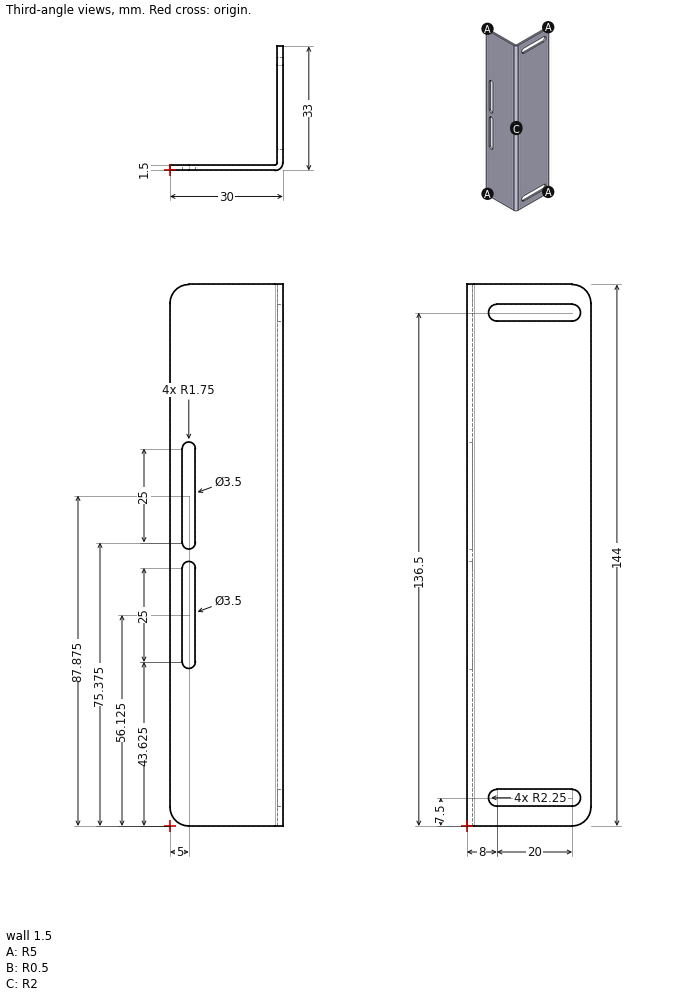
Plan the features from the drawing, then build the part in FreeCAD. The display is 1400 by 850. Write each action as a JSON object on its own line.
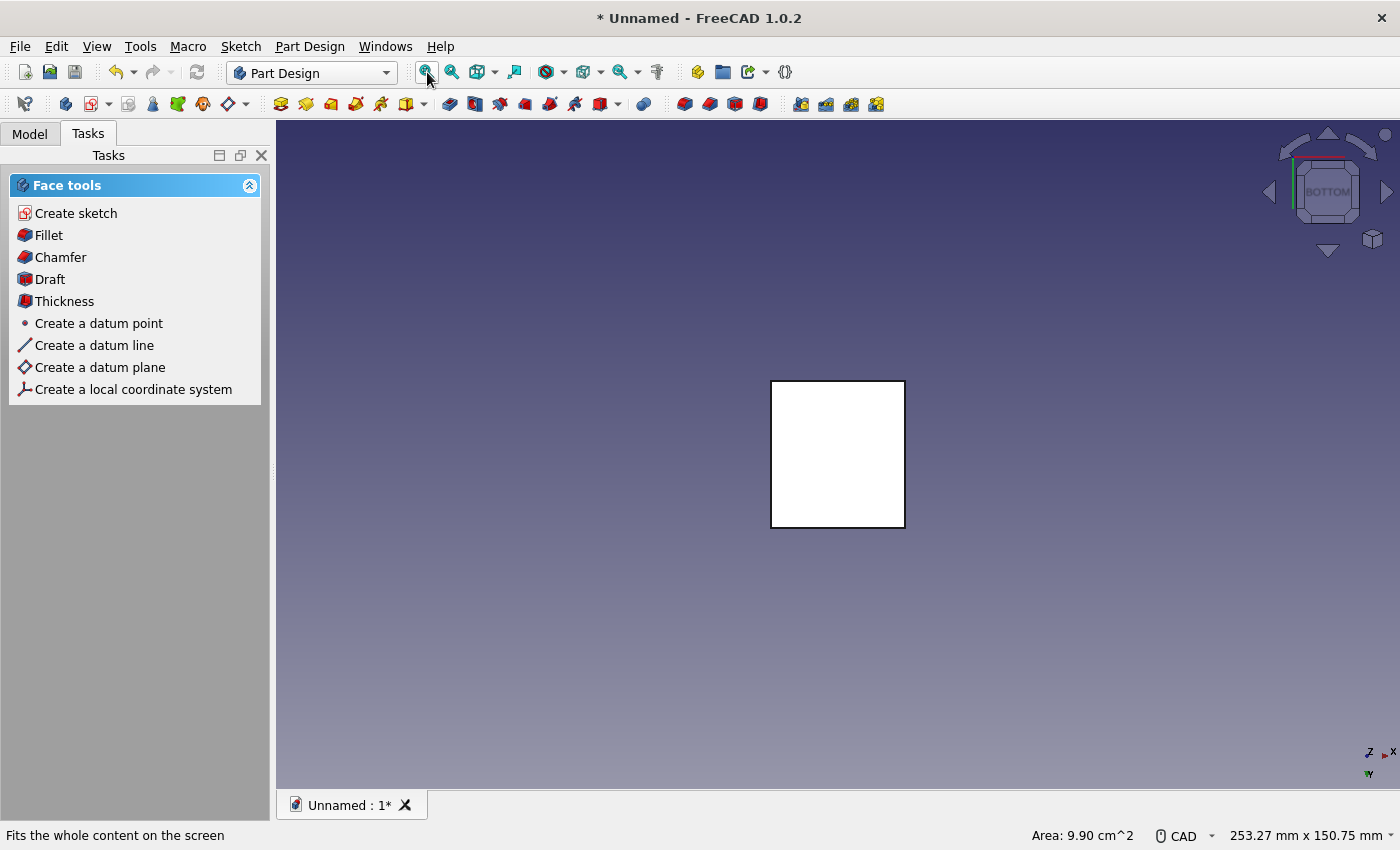
{"action": "left_click", "coordinate": [838, 453], "text": "ctrl"}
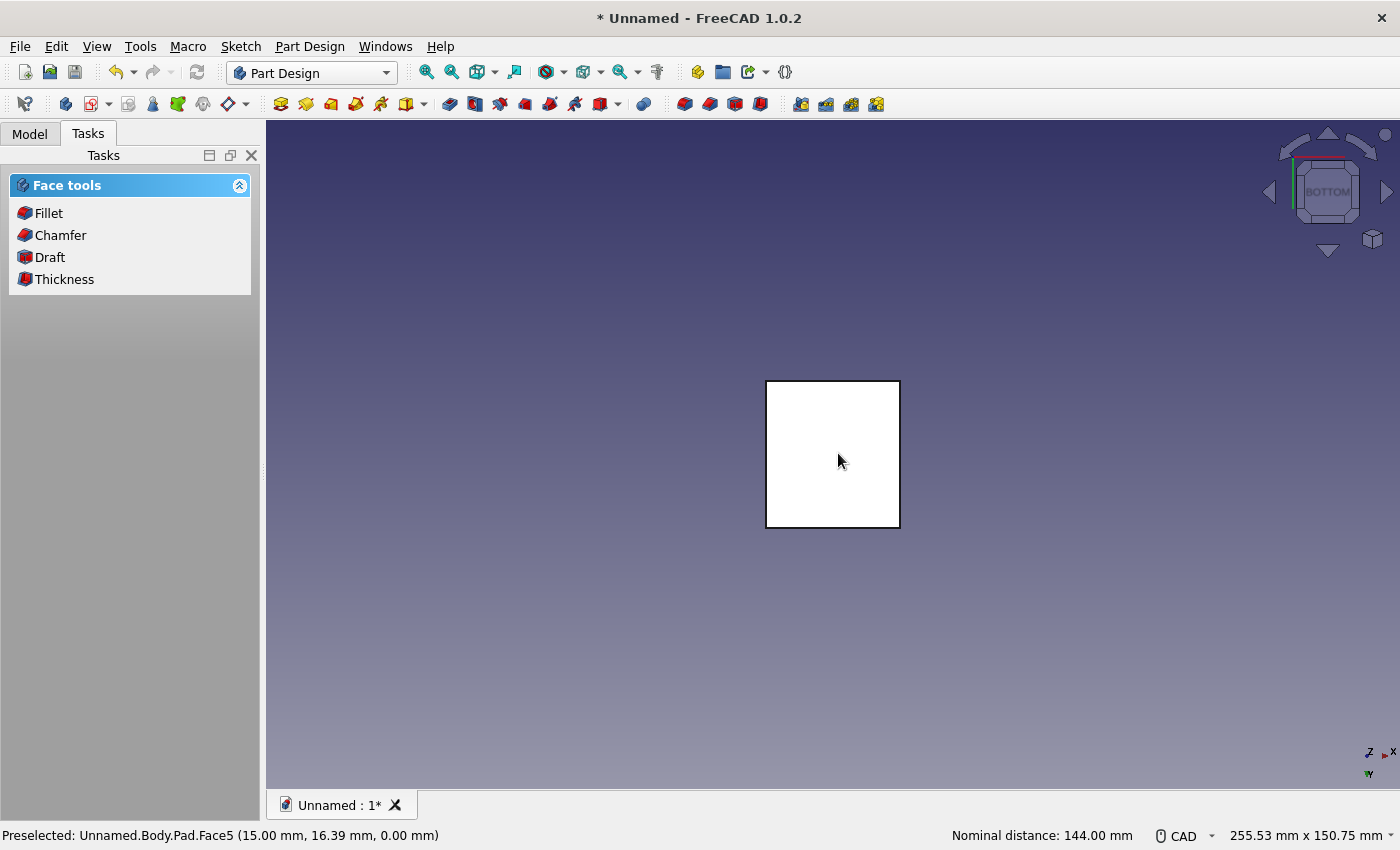
{"action": "key", "text": "4"}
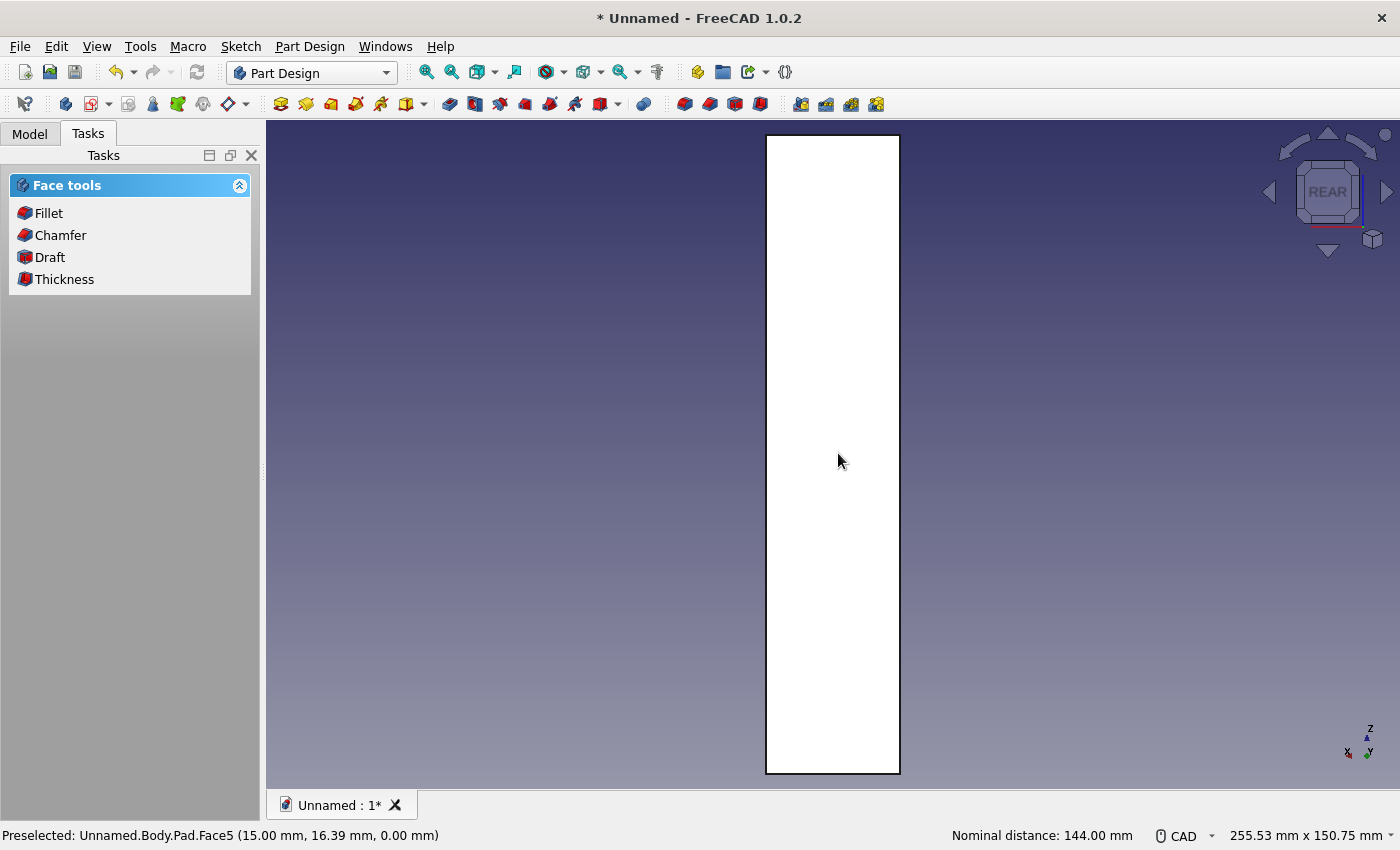
{"action": "left_click", "coordinate": [833, 271], "text": "ctrl"}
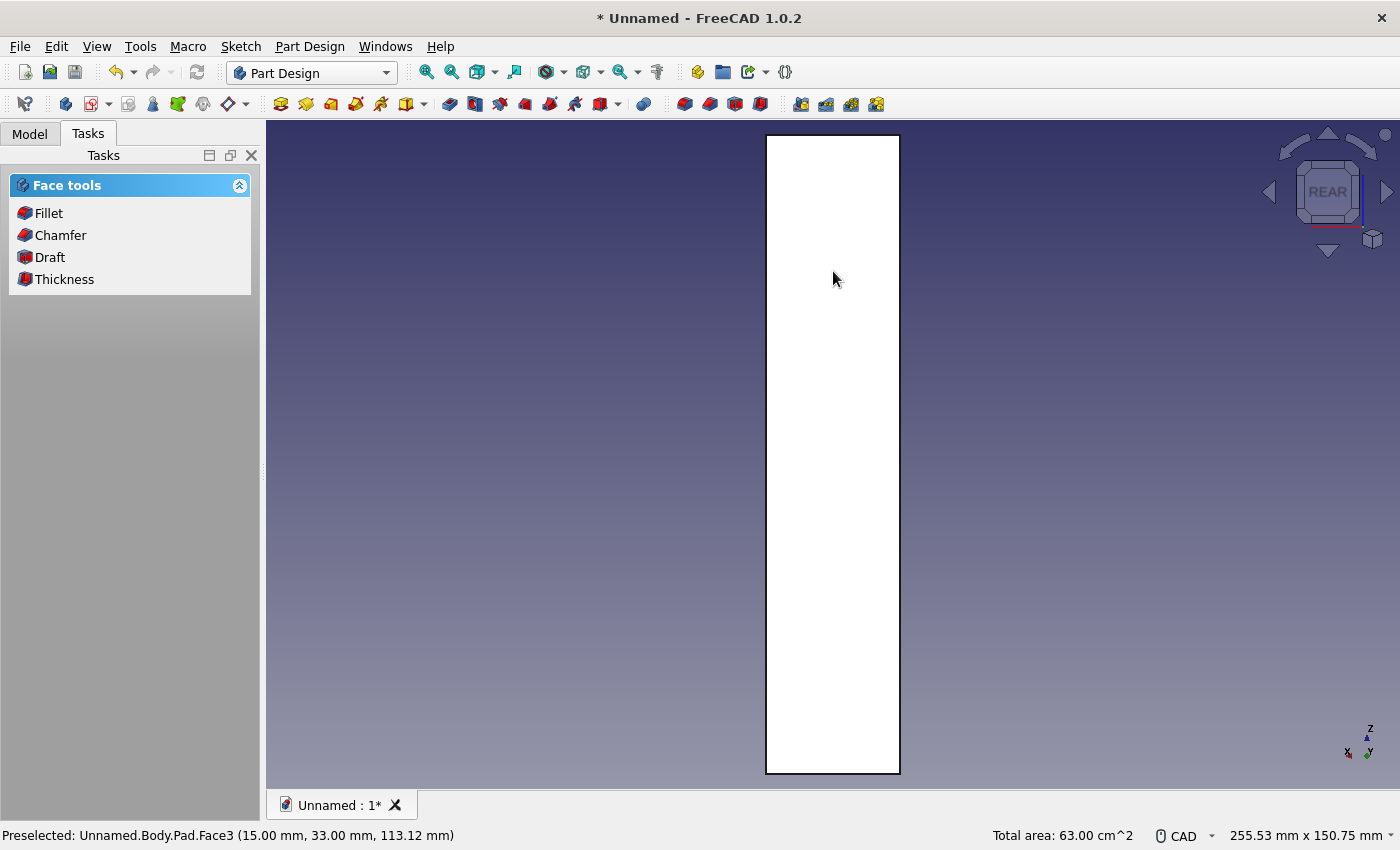
{"action": "key", "text": "6"}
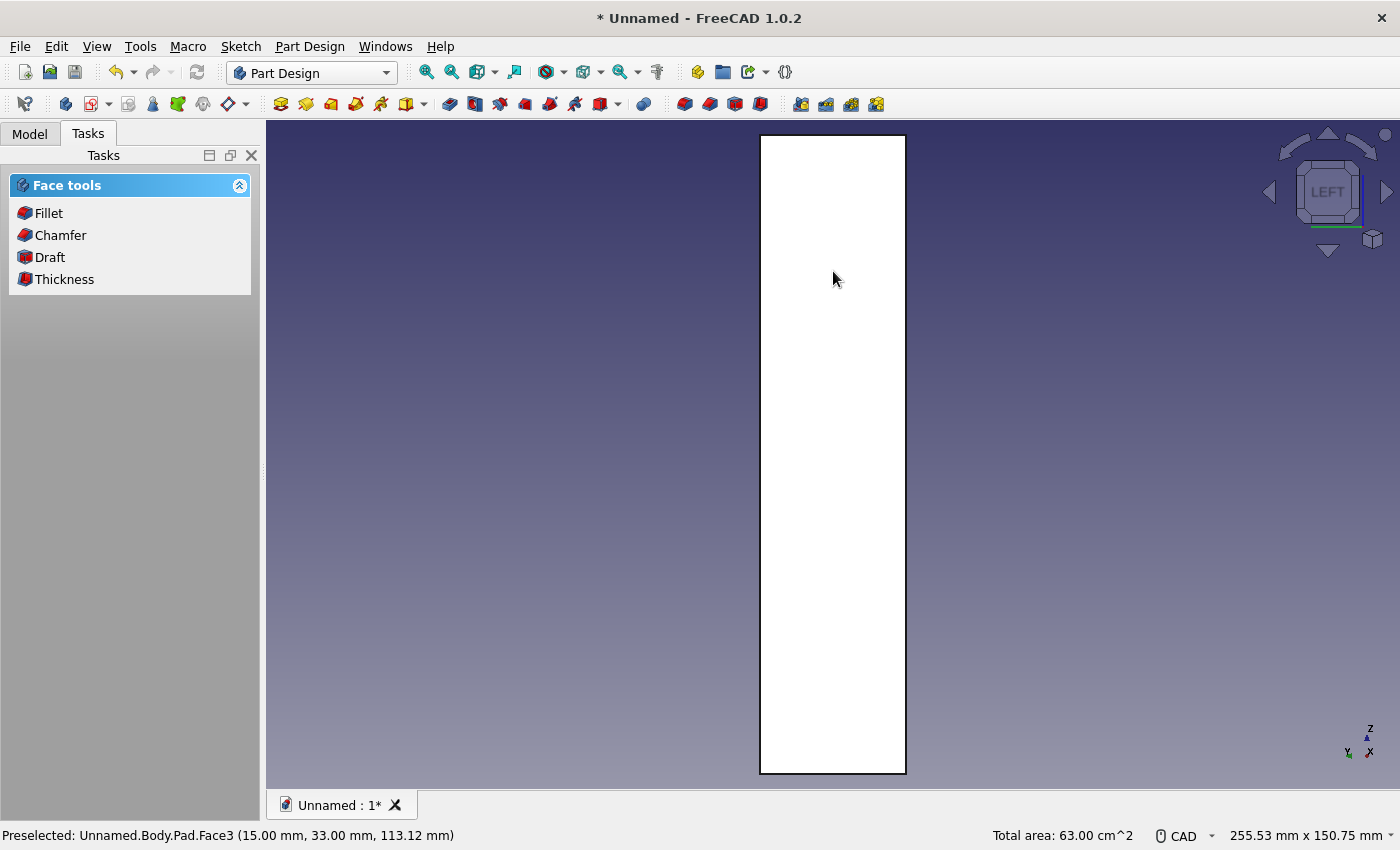
{"action": "left_click", "coordinate": [833, 271], "text": "ctrl"}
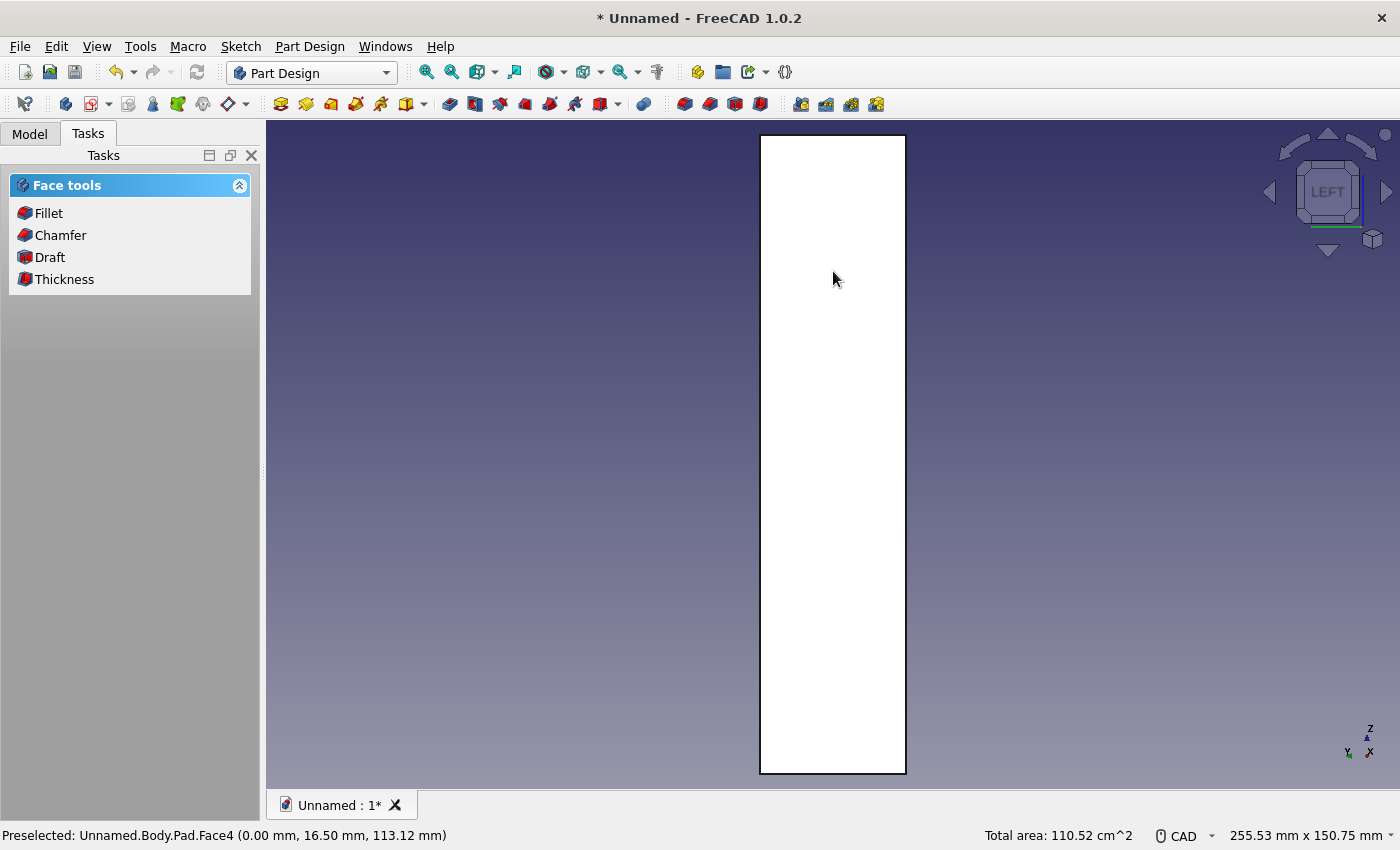
{"action": "left_click", "coordinate": [760, 104]}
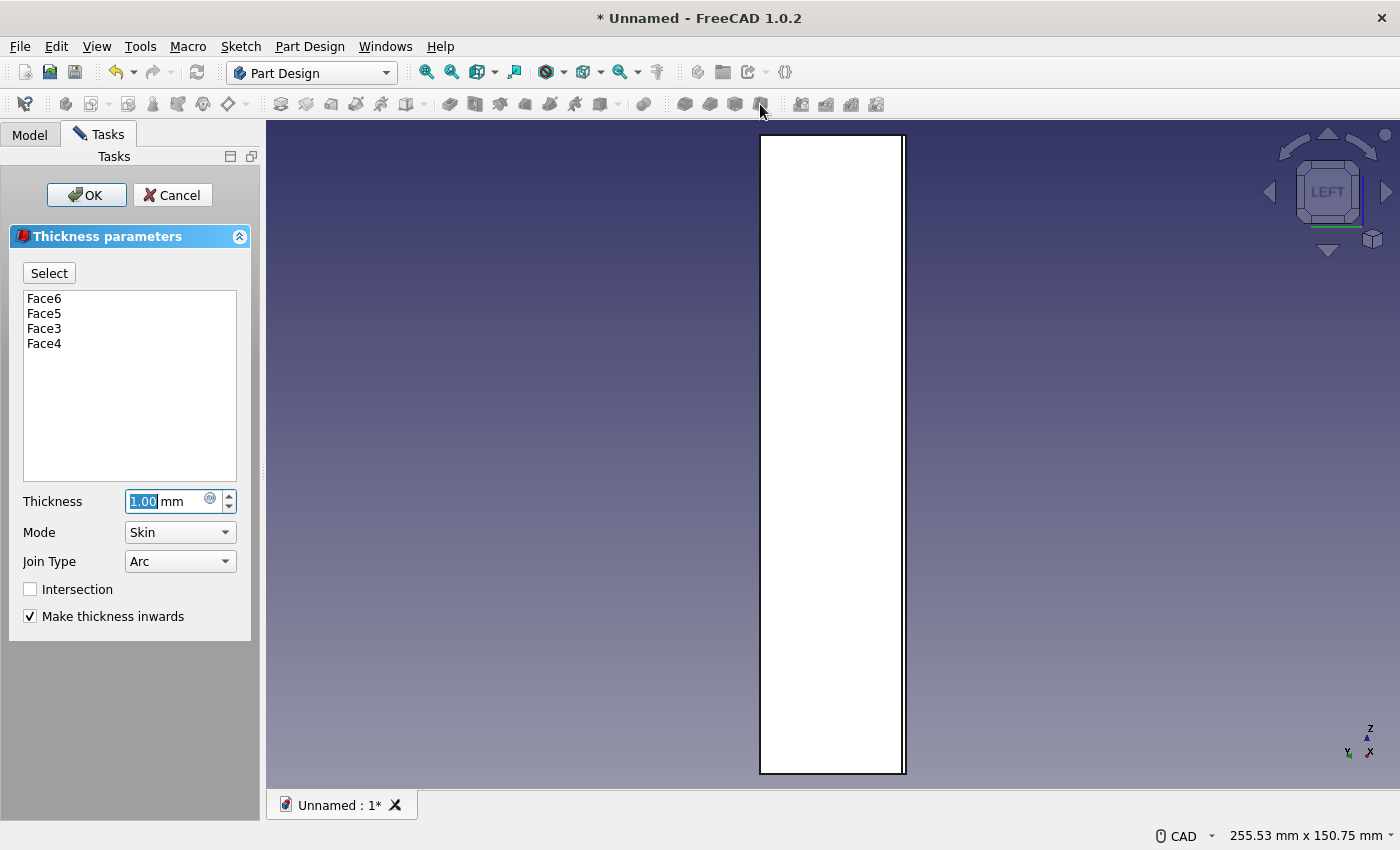
{"action": "type", "text": "1.5"}
{"action": "key", "text": "Tab"}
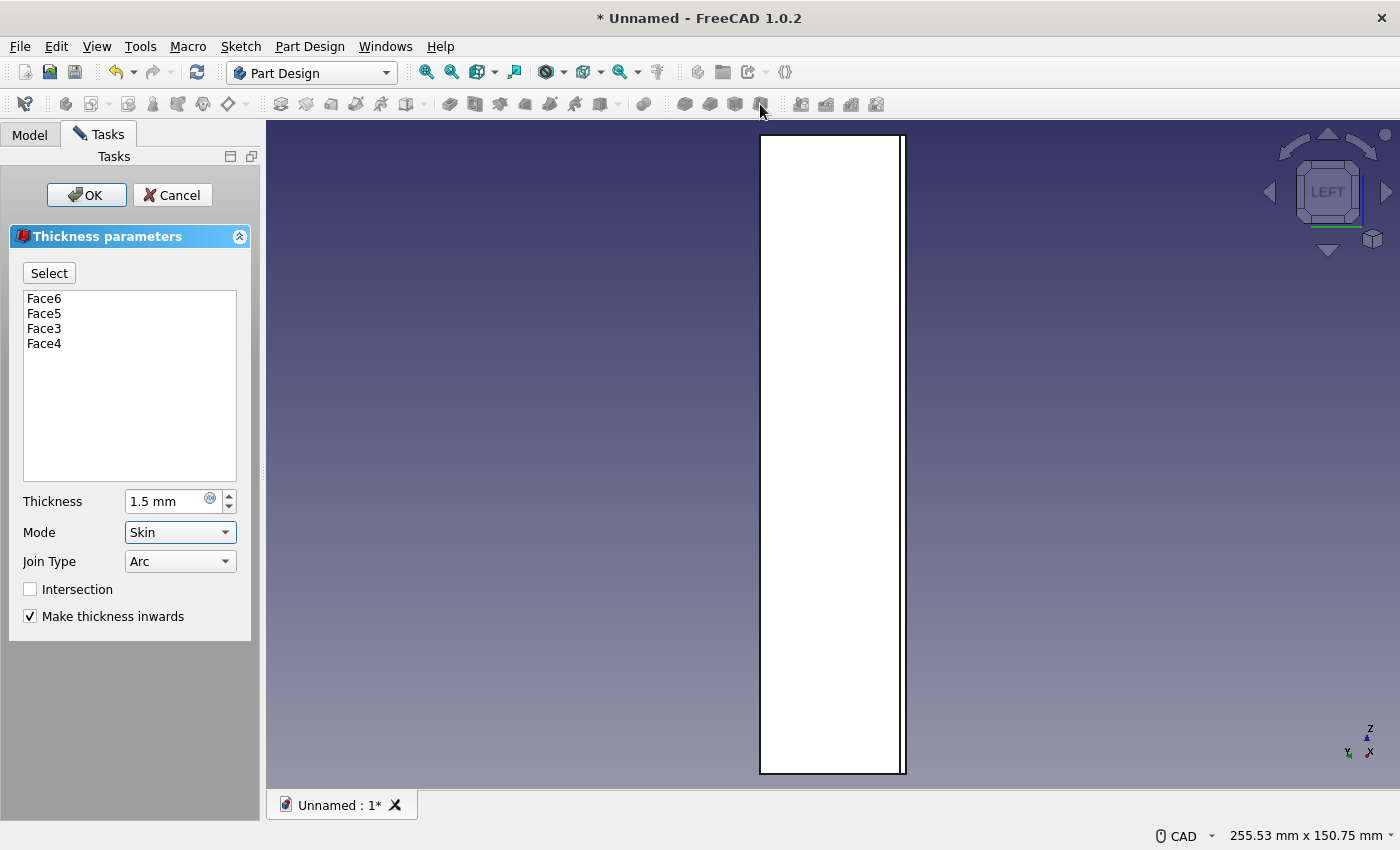
{"action": "left_click", "coordinate": [181, 562]}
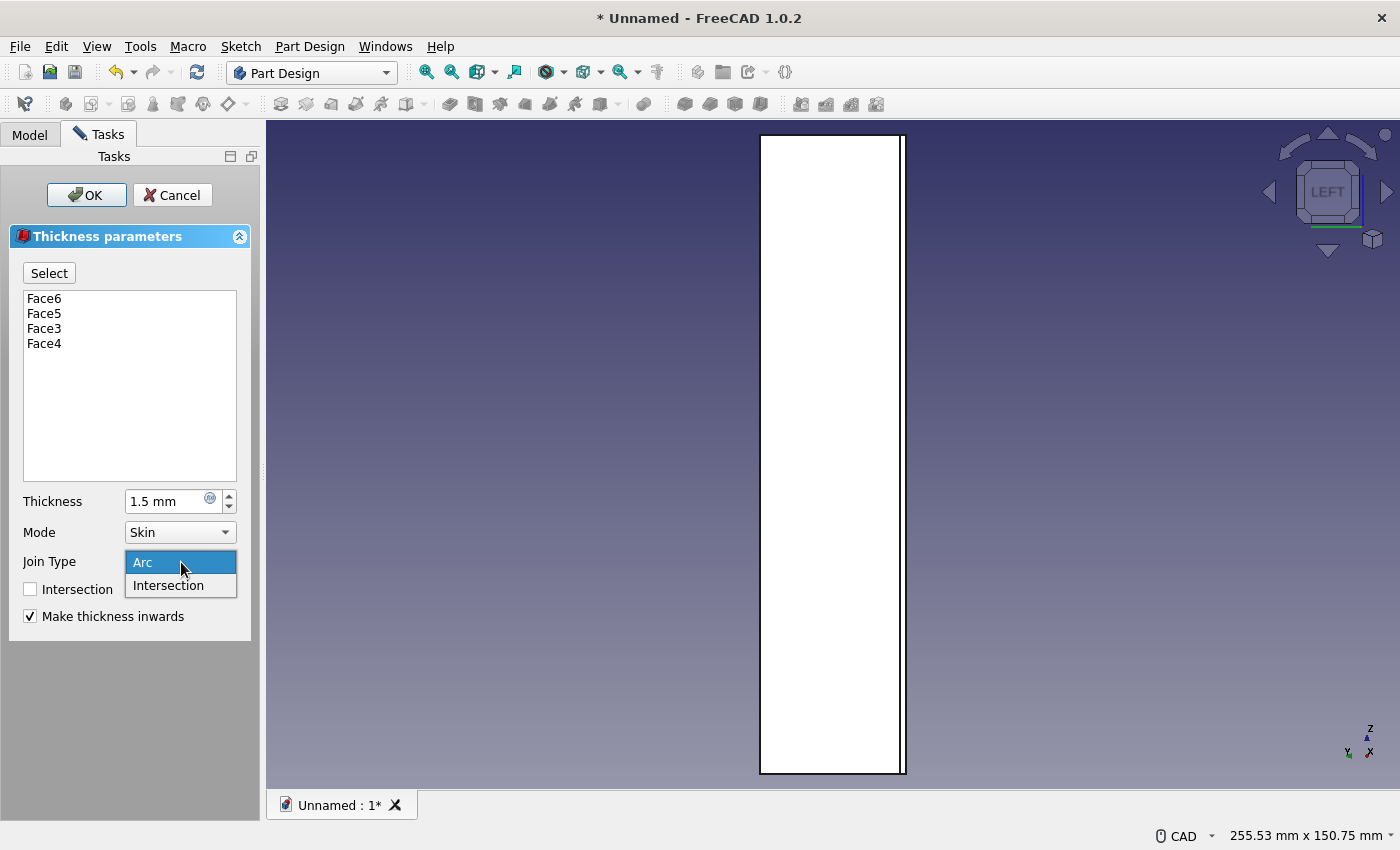
{"action": "left_click", "coordinate": [179, 586]}